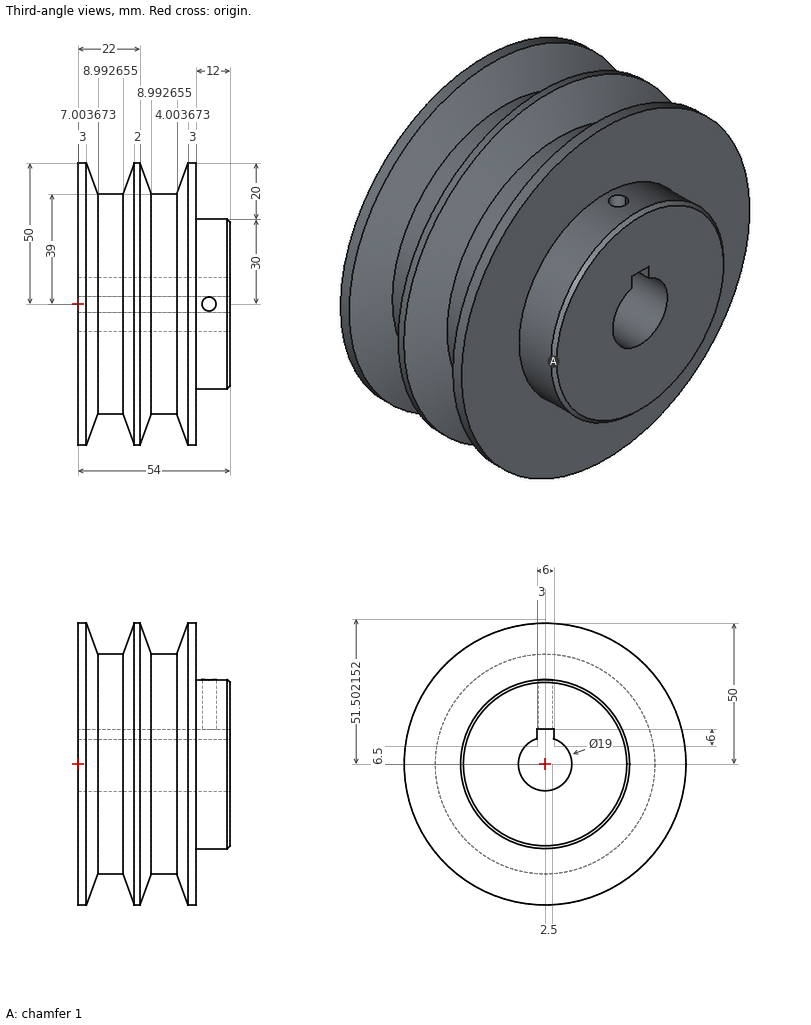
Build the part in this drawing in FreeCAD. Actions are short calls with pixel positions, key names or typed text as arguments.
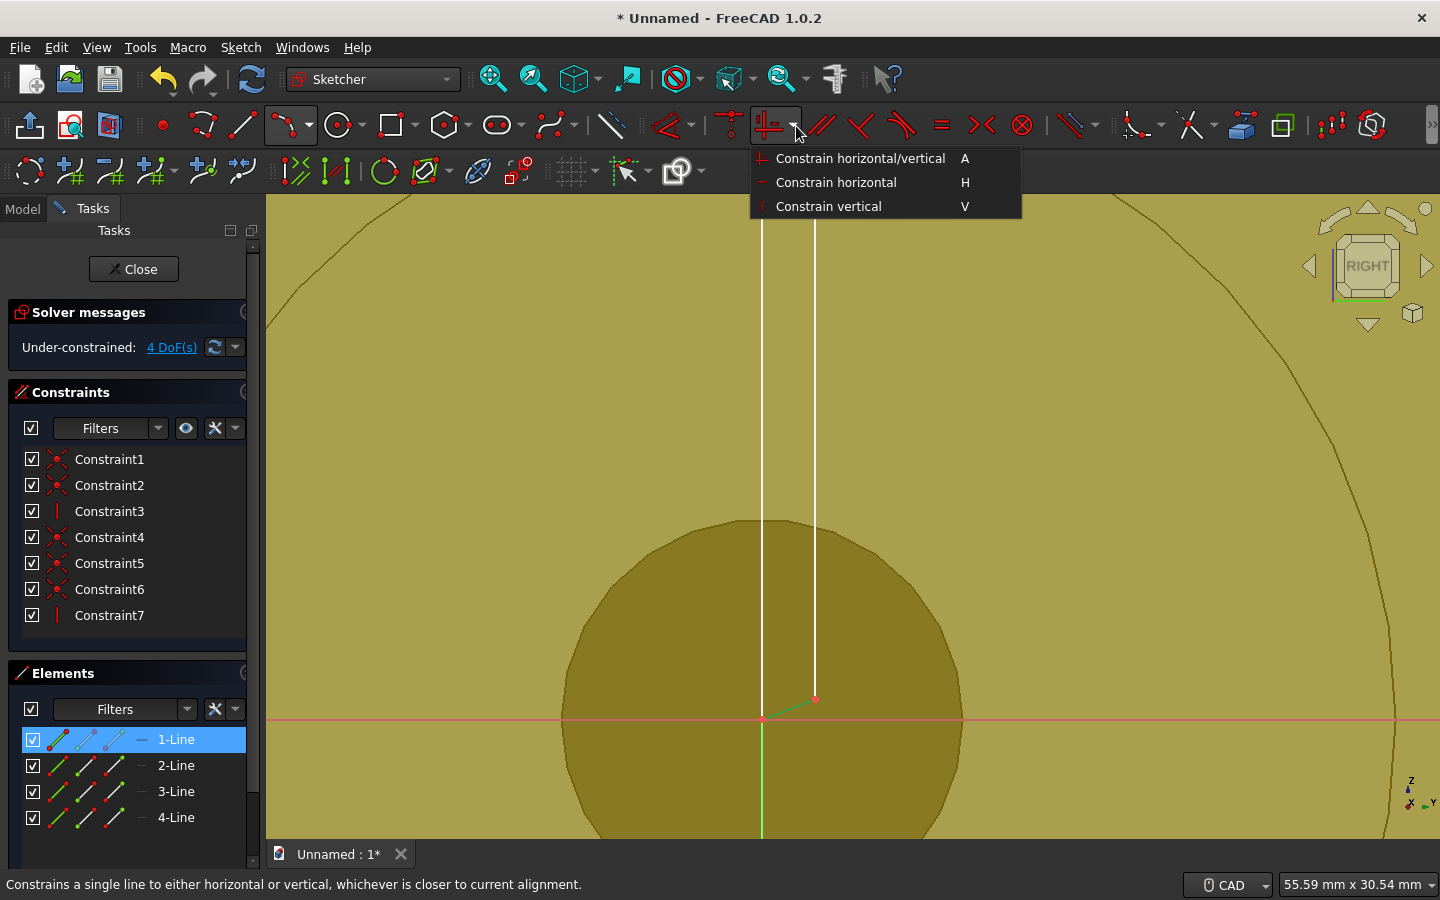
click(886, 182)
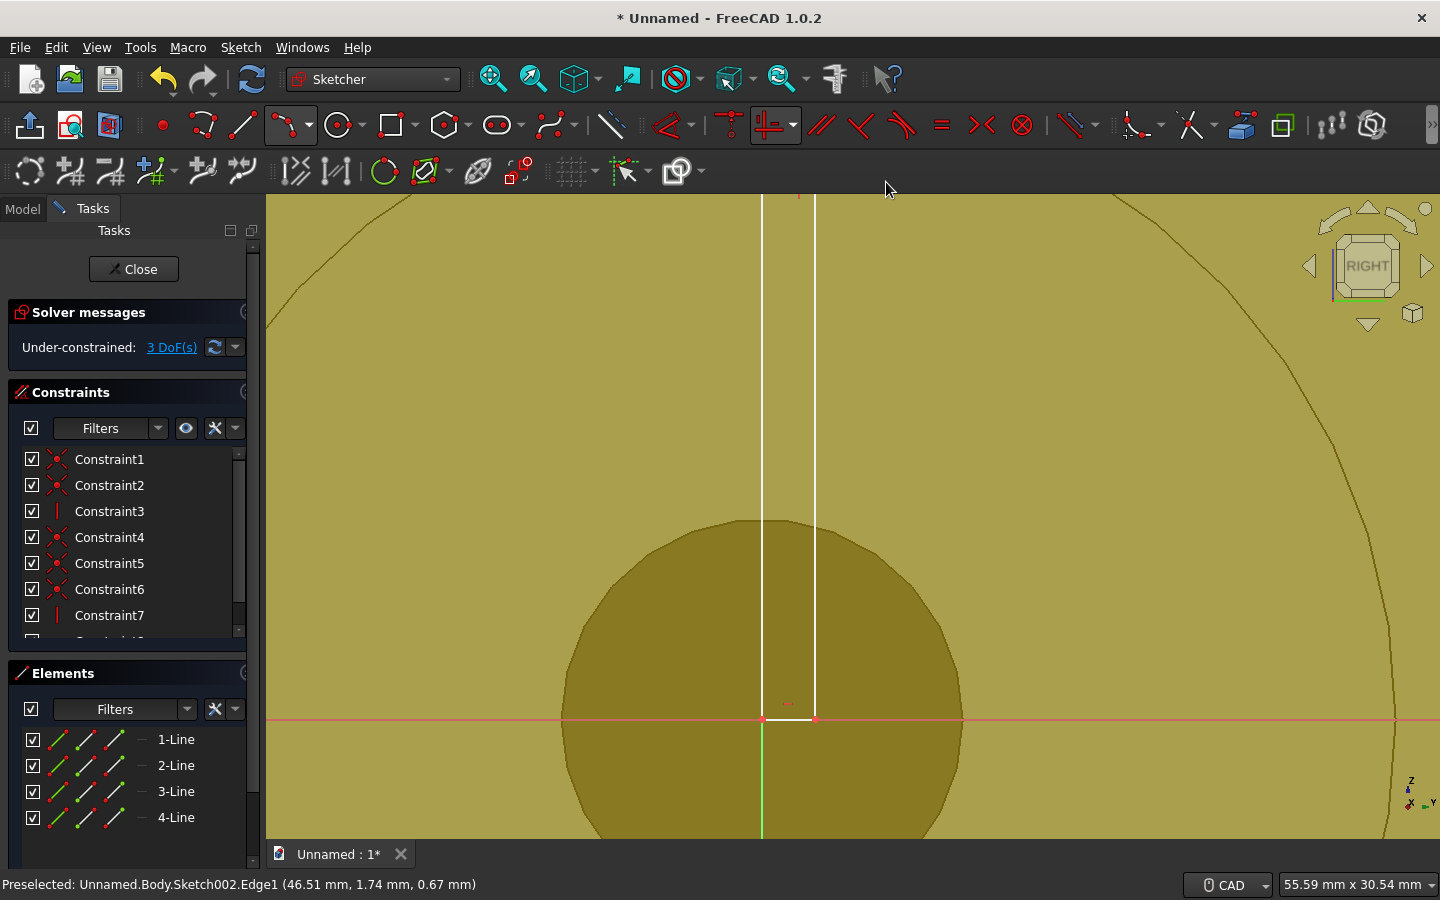
click(666, 126)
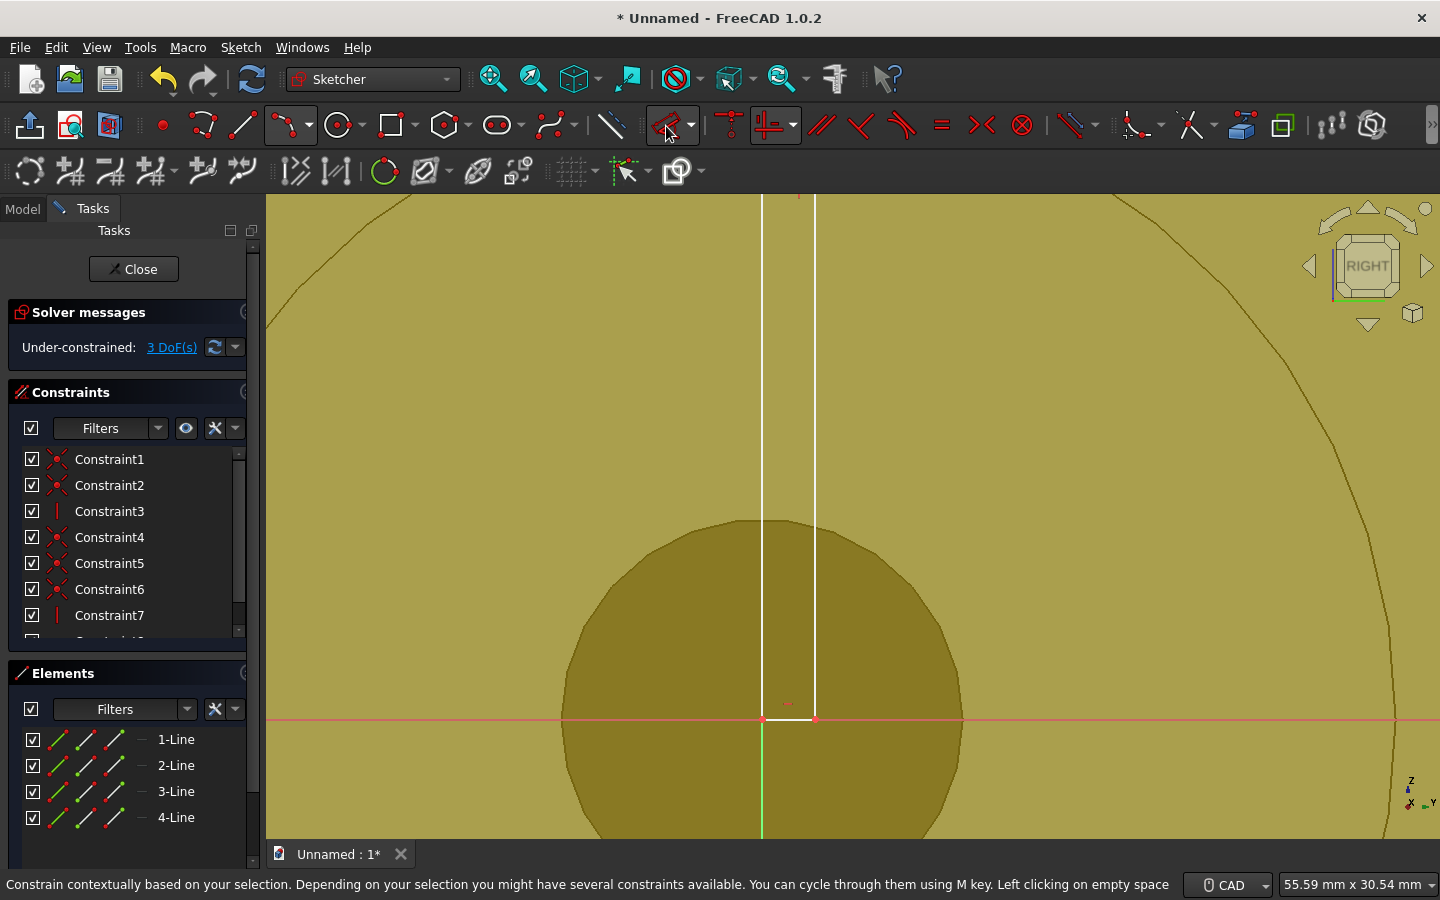
click(815, 404)
click(849, 471)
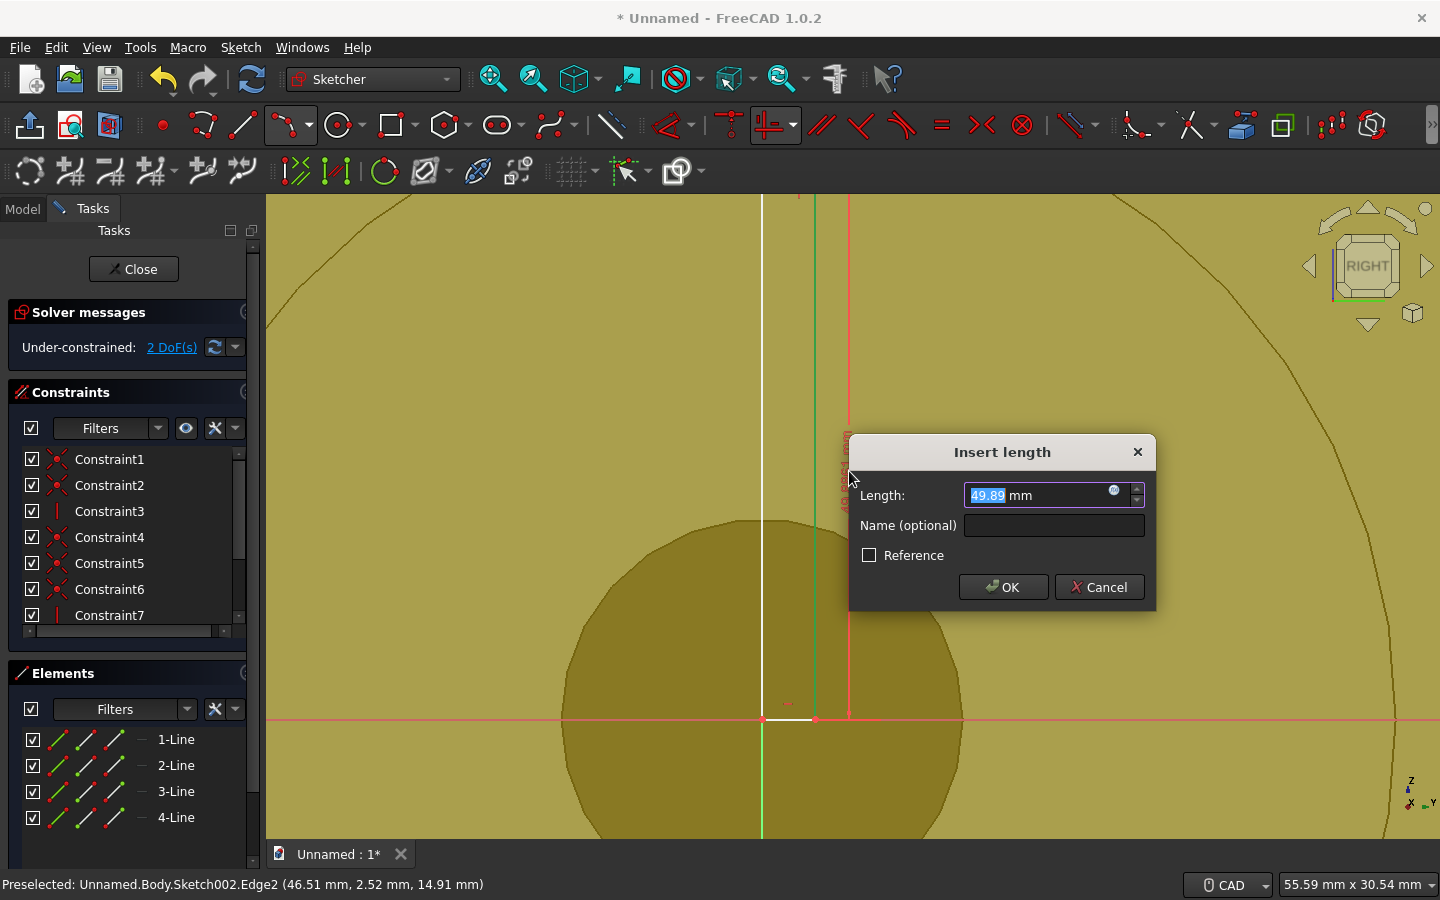
text(50)
key(Return)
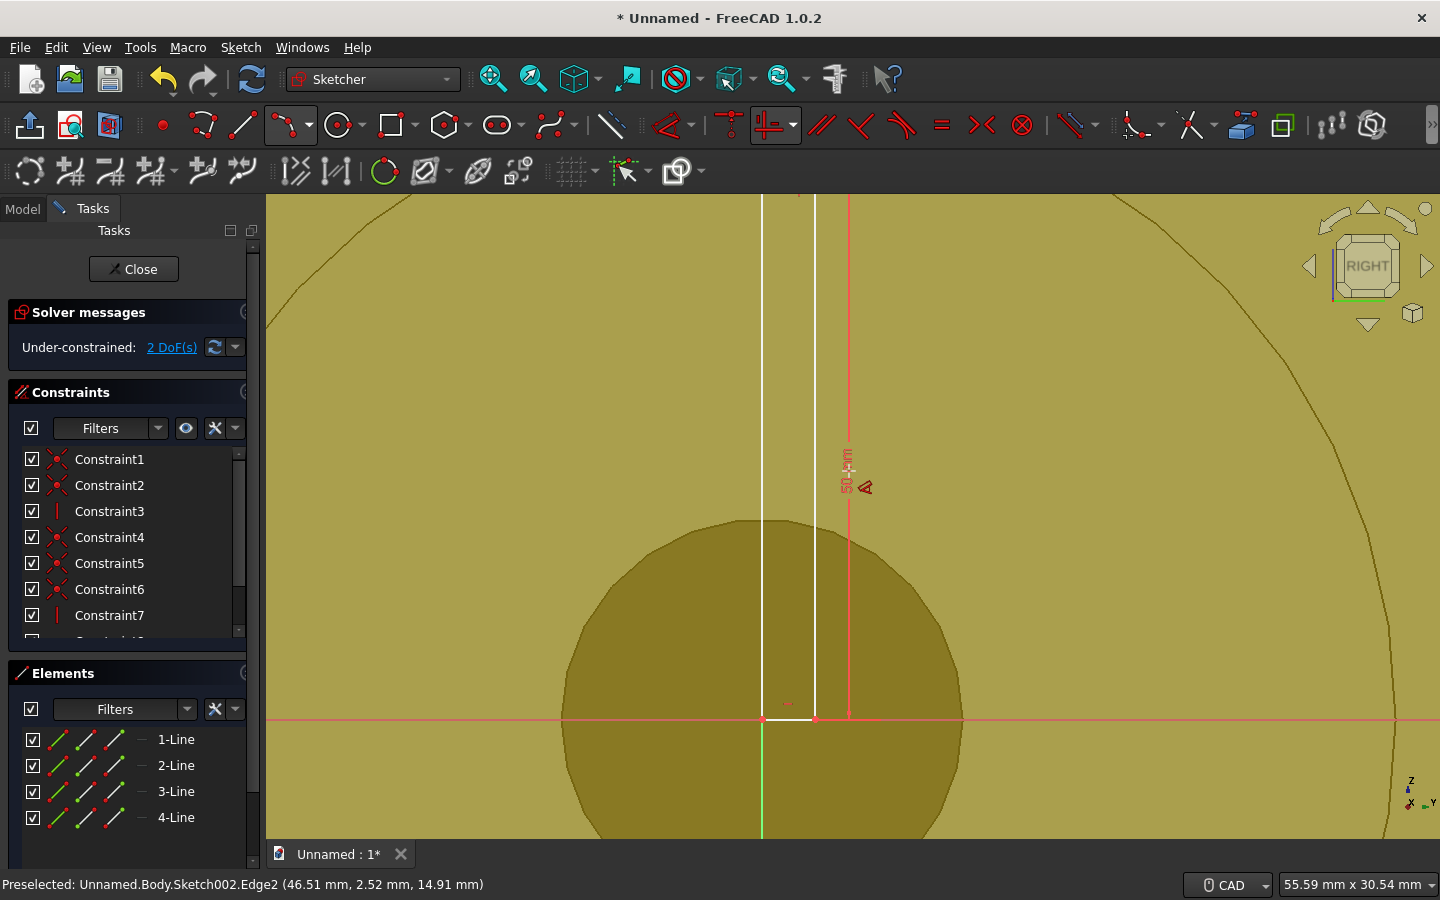
click(778, 720)
click(789, 754)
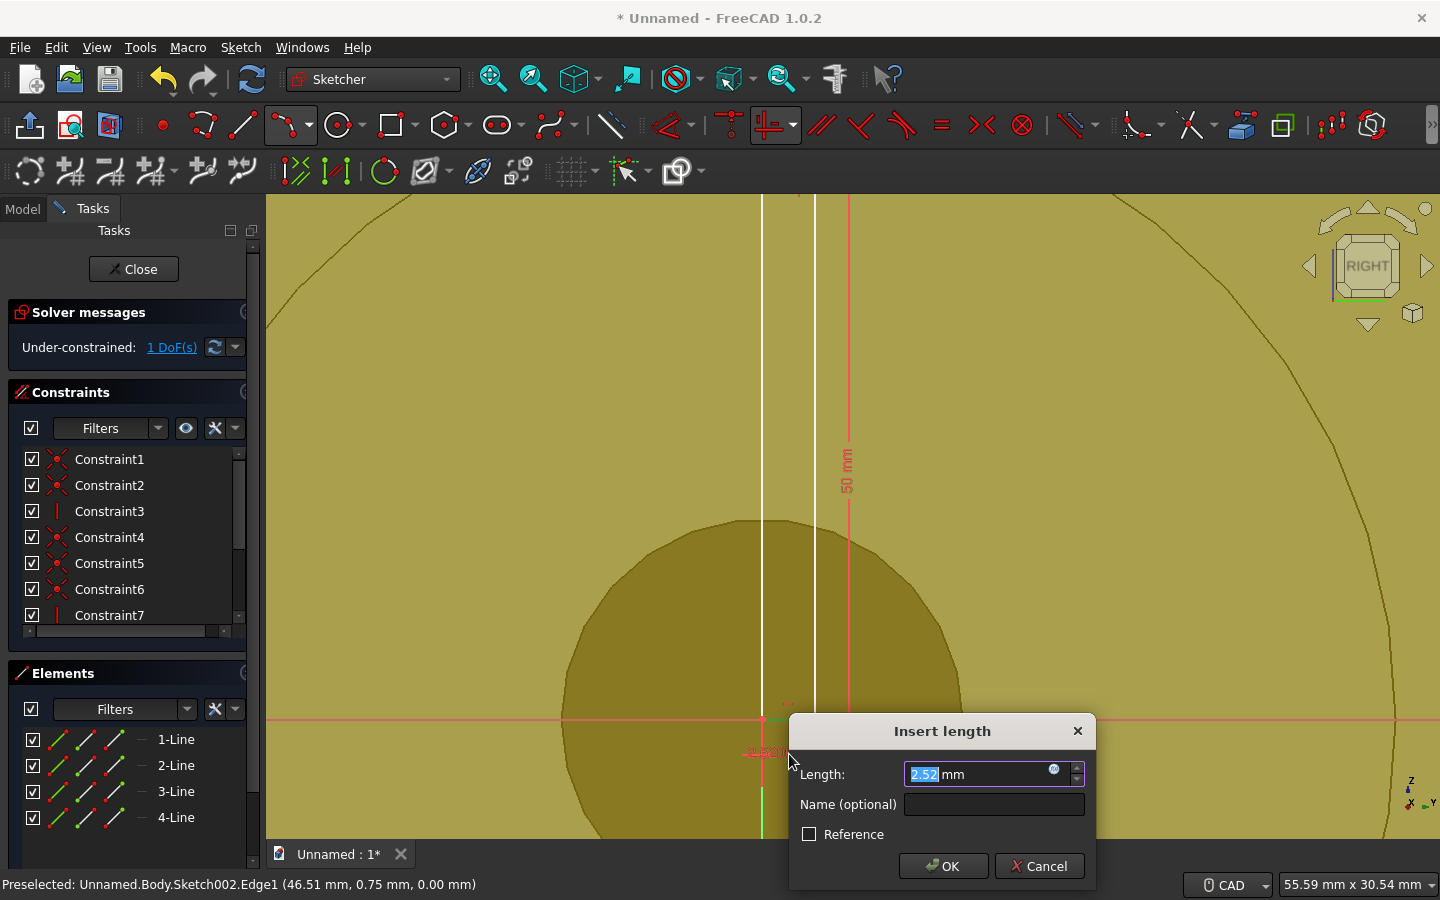
text(2.5)
key(Return)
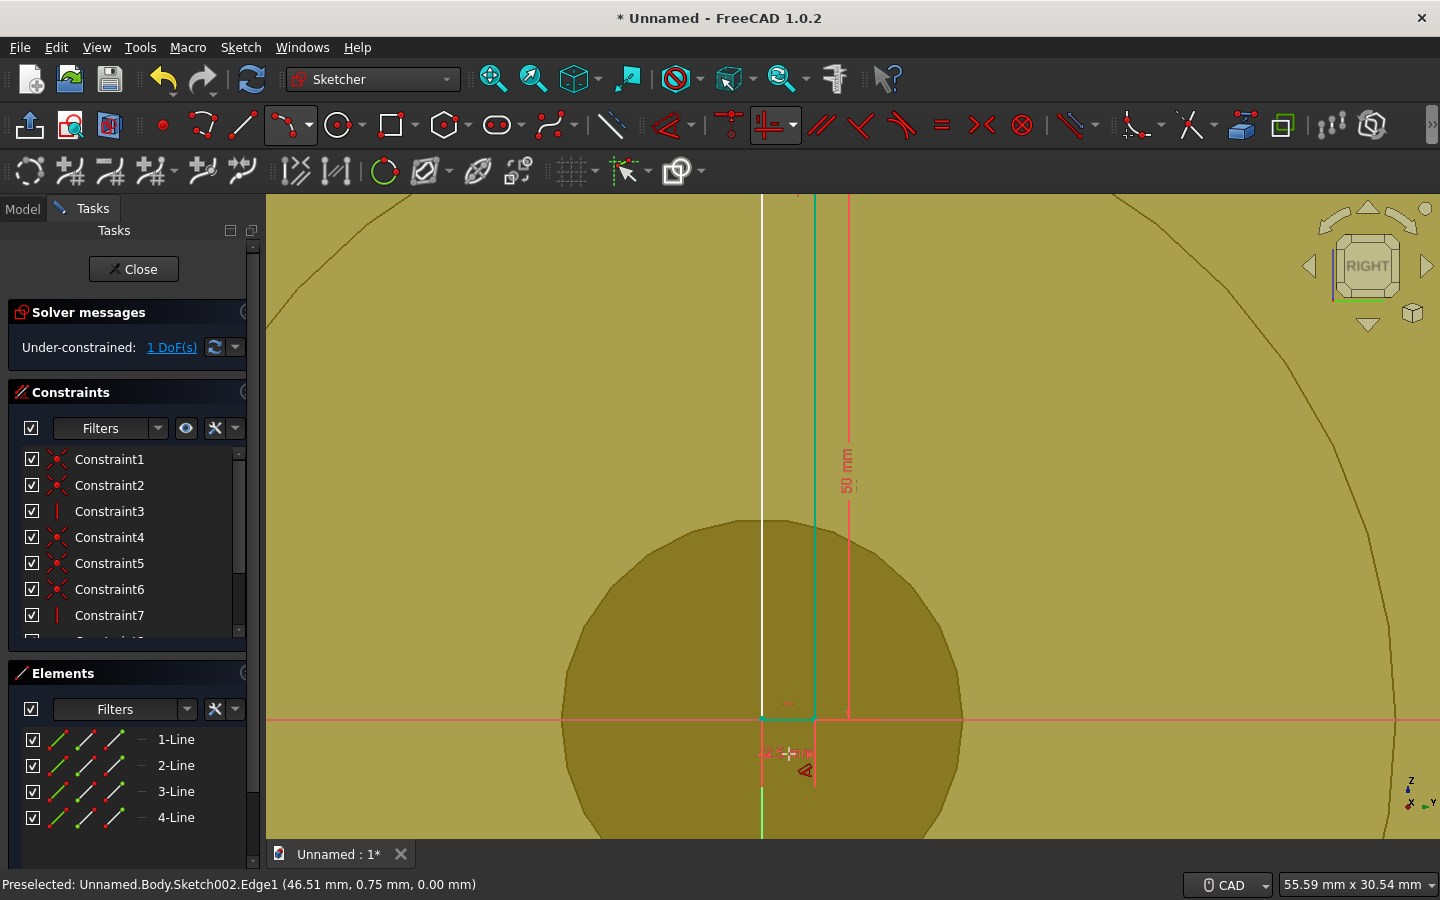
click(762, 394)
click(728, 471)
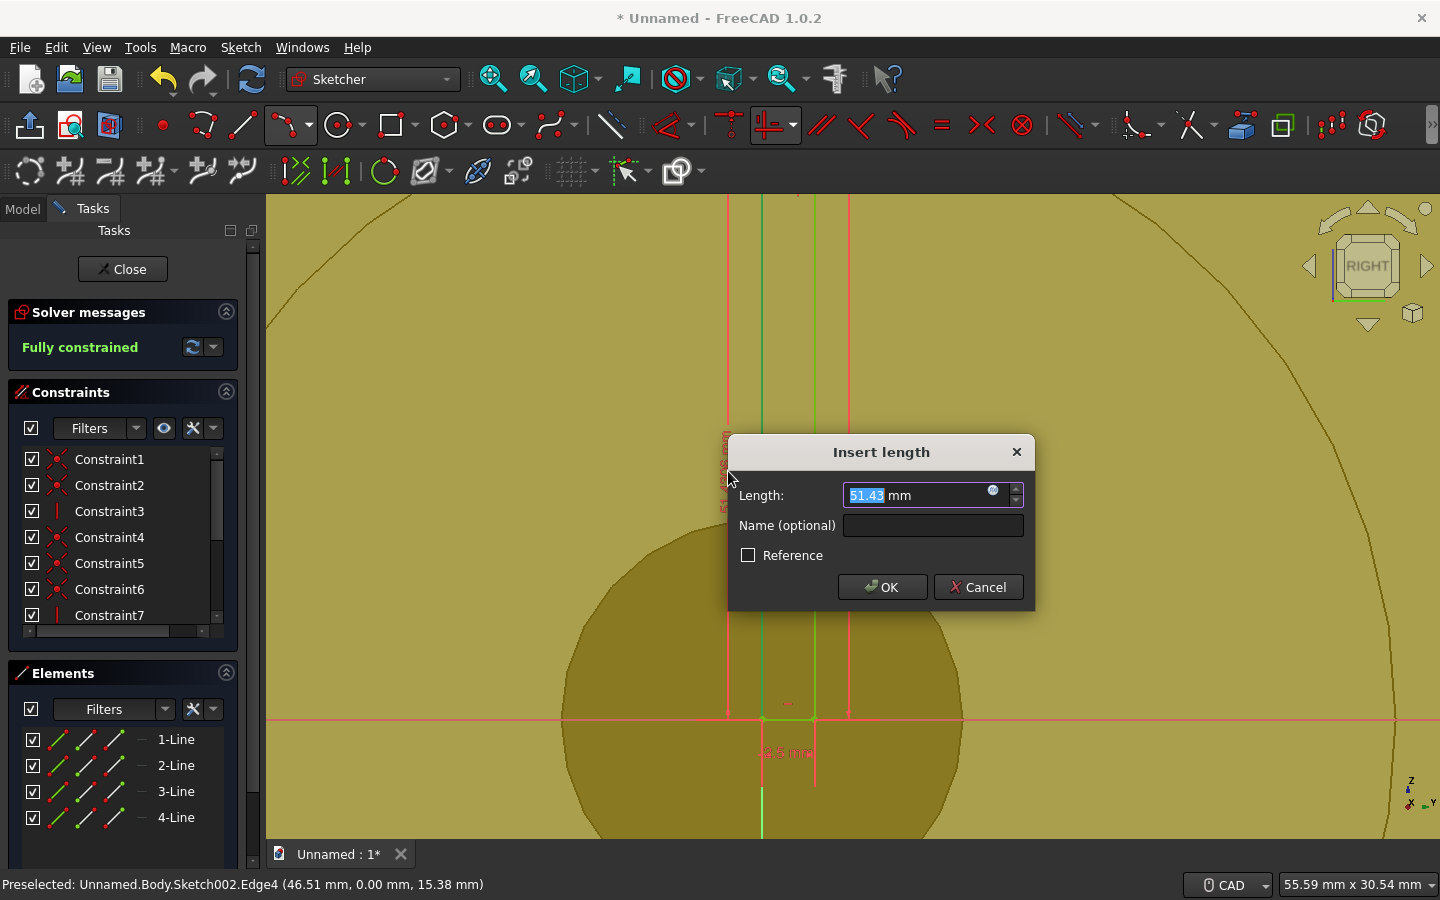
text(51.502152)
key(Return)
key(Escape)